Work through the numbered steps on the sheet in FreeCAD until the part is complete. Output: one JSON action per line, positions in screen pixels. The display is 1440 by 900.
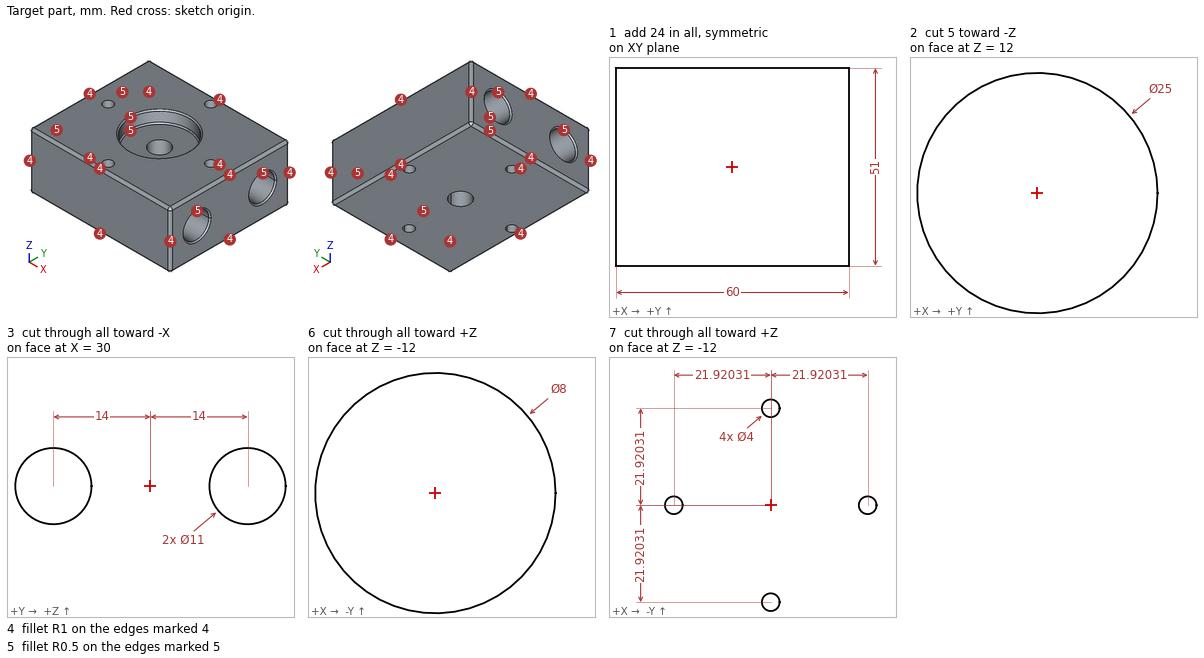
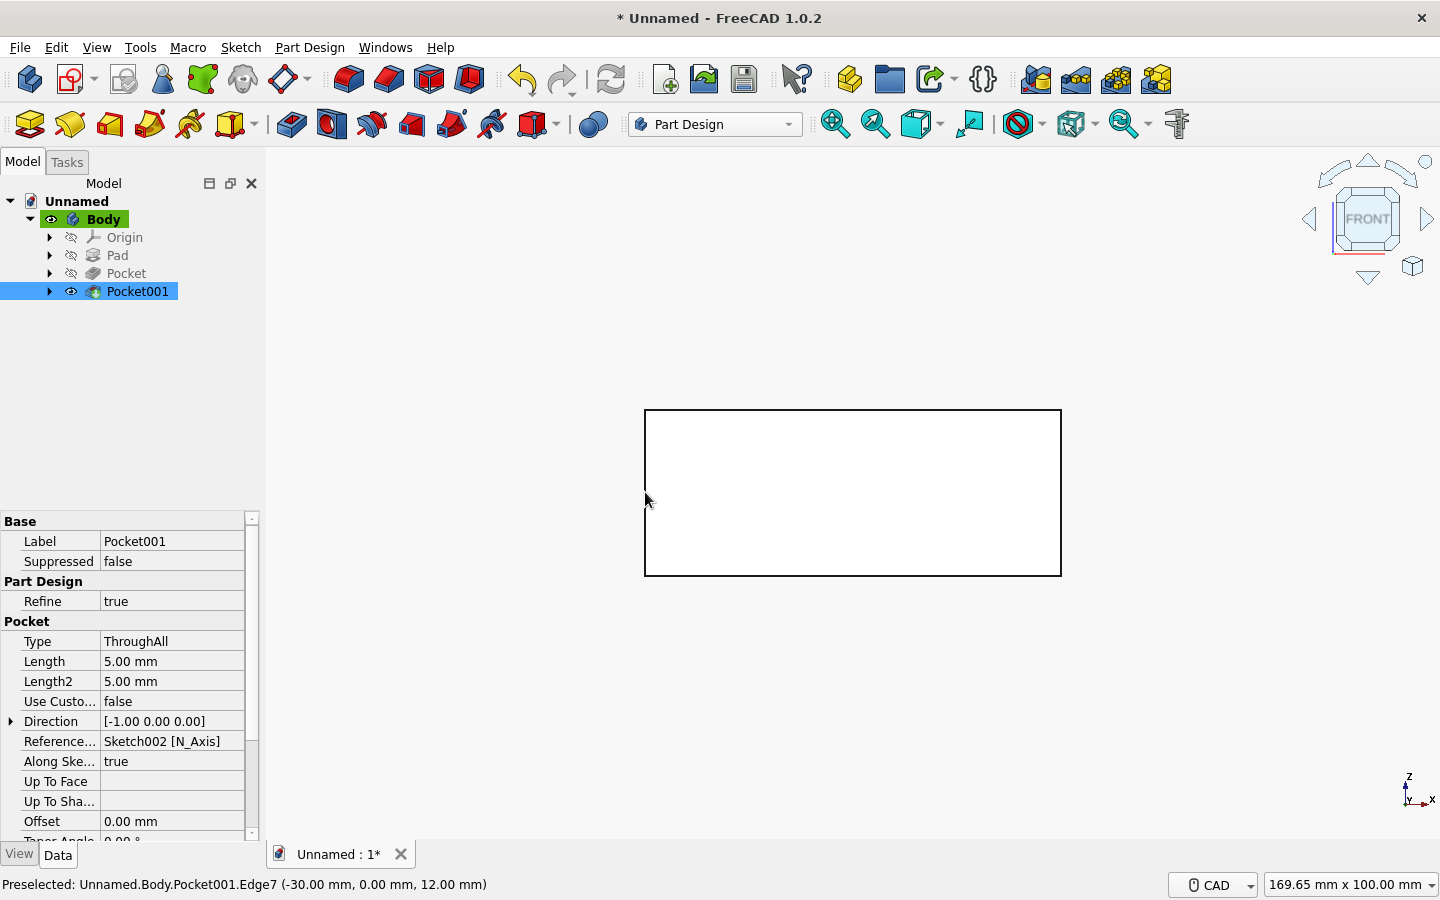
{"action": "key", "text": "v f"}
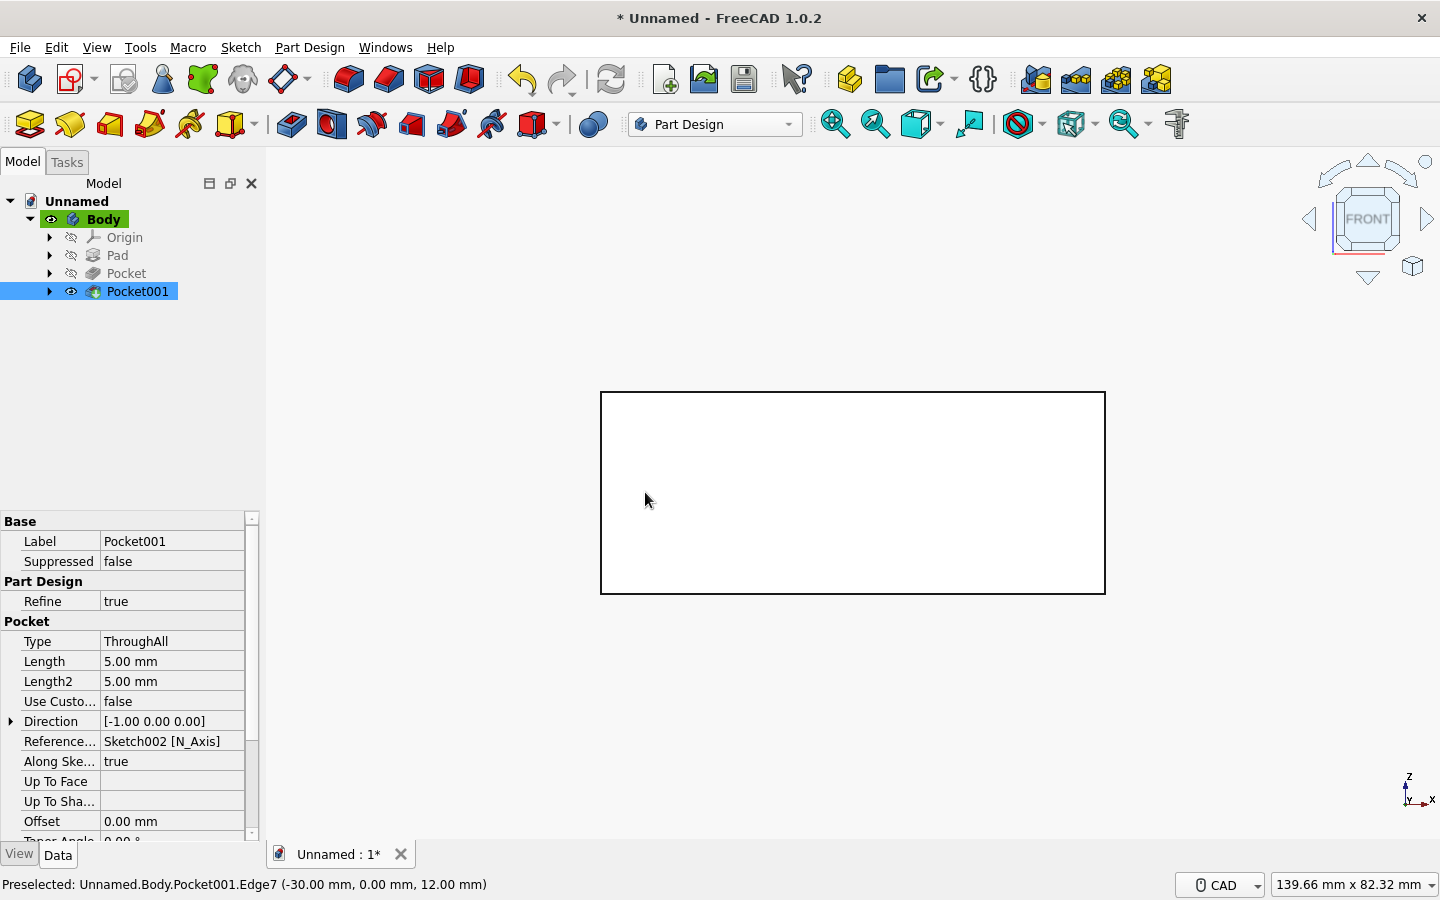
{"action": "key", "text": "3"}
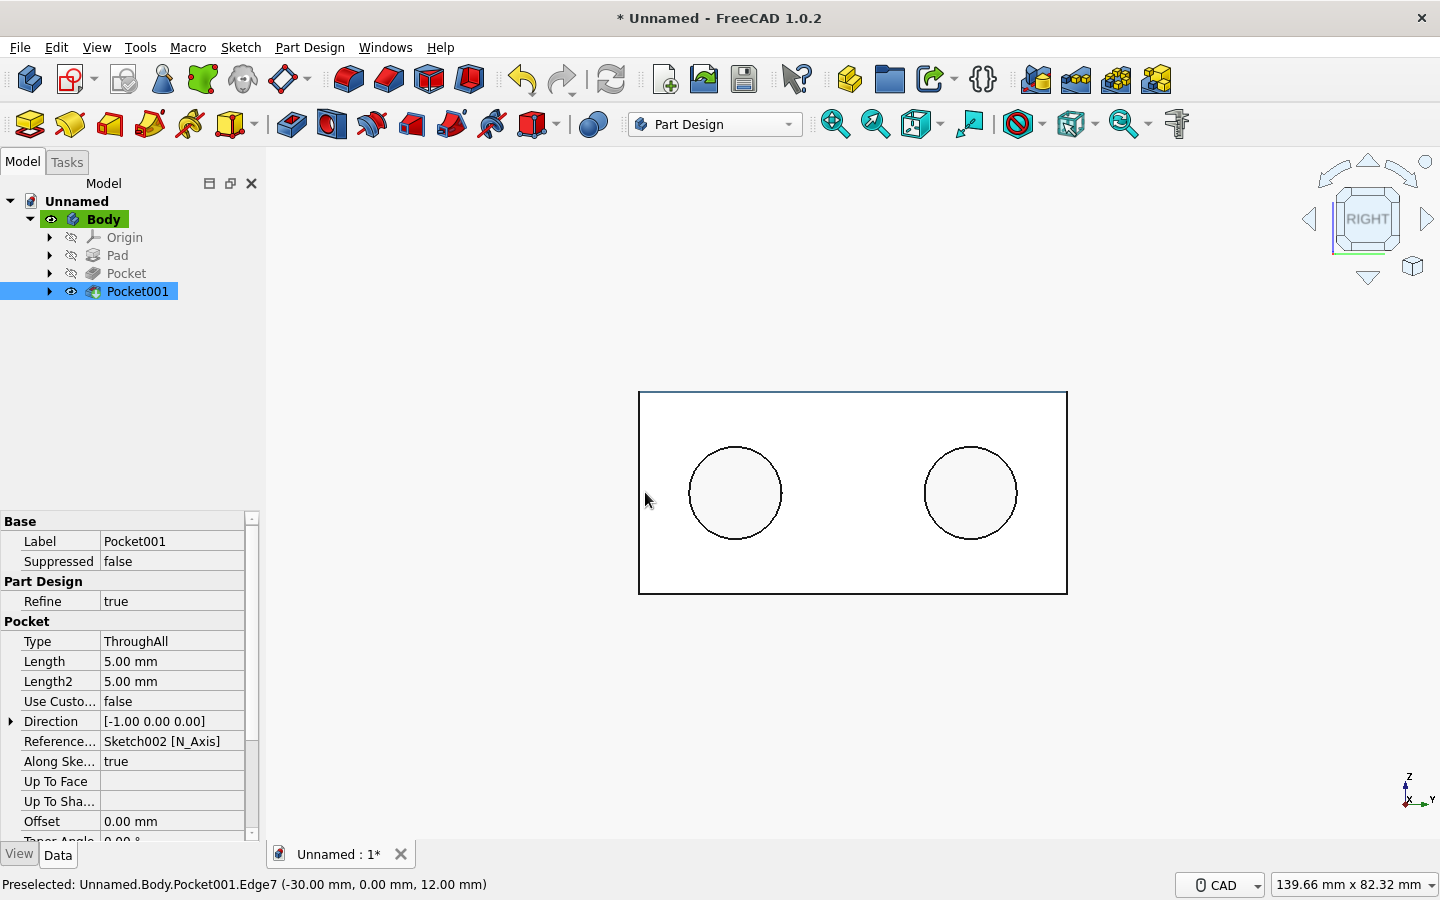
{"action": "key", "text": "v f"}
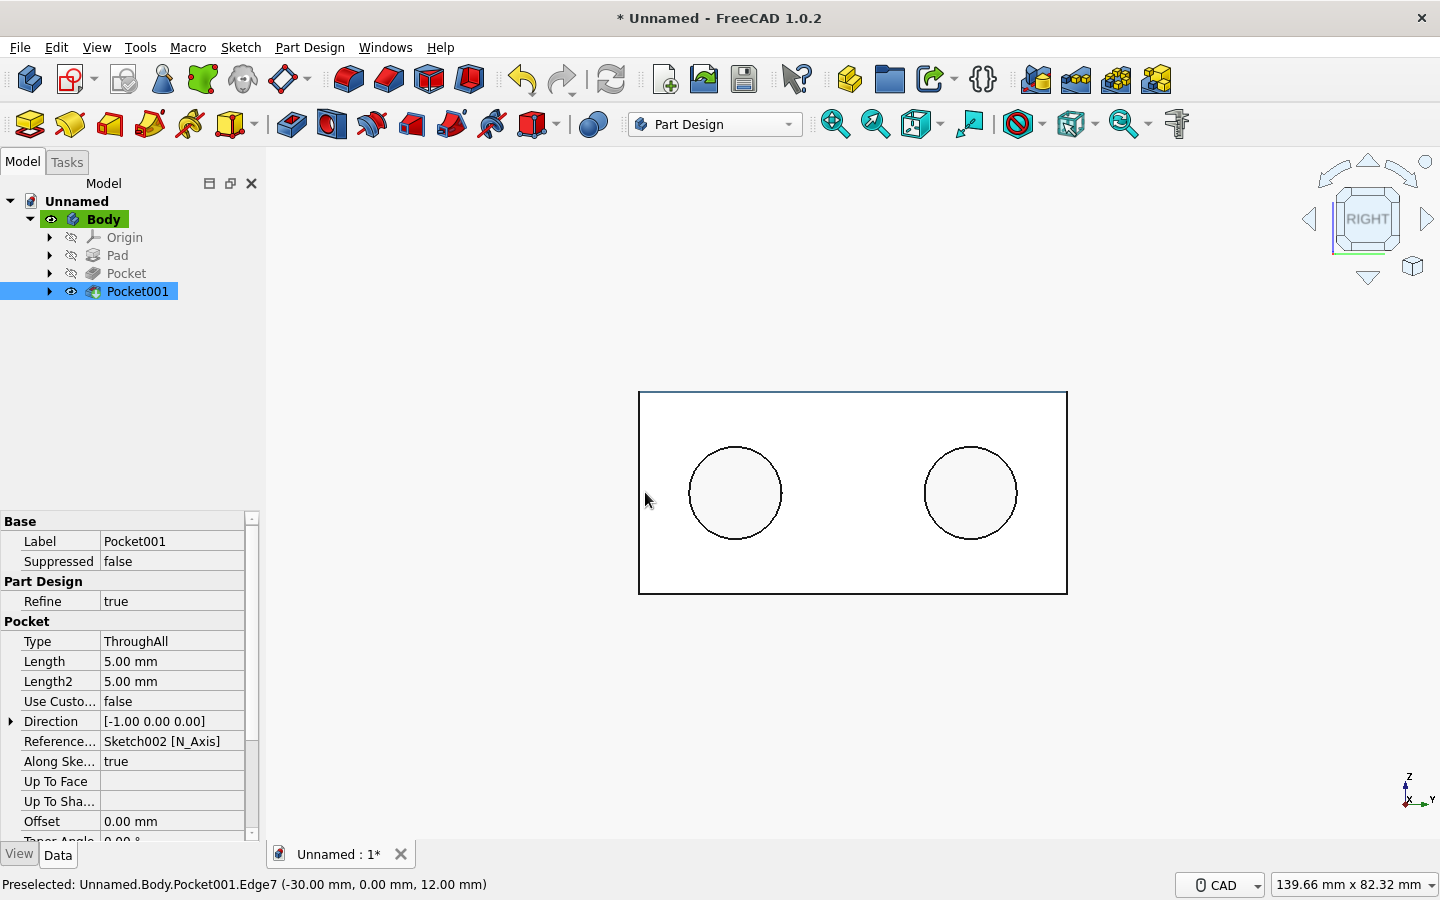
{"action": "key", "text": "5"}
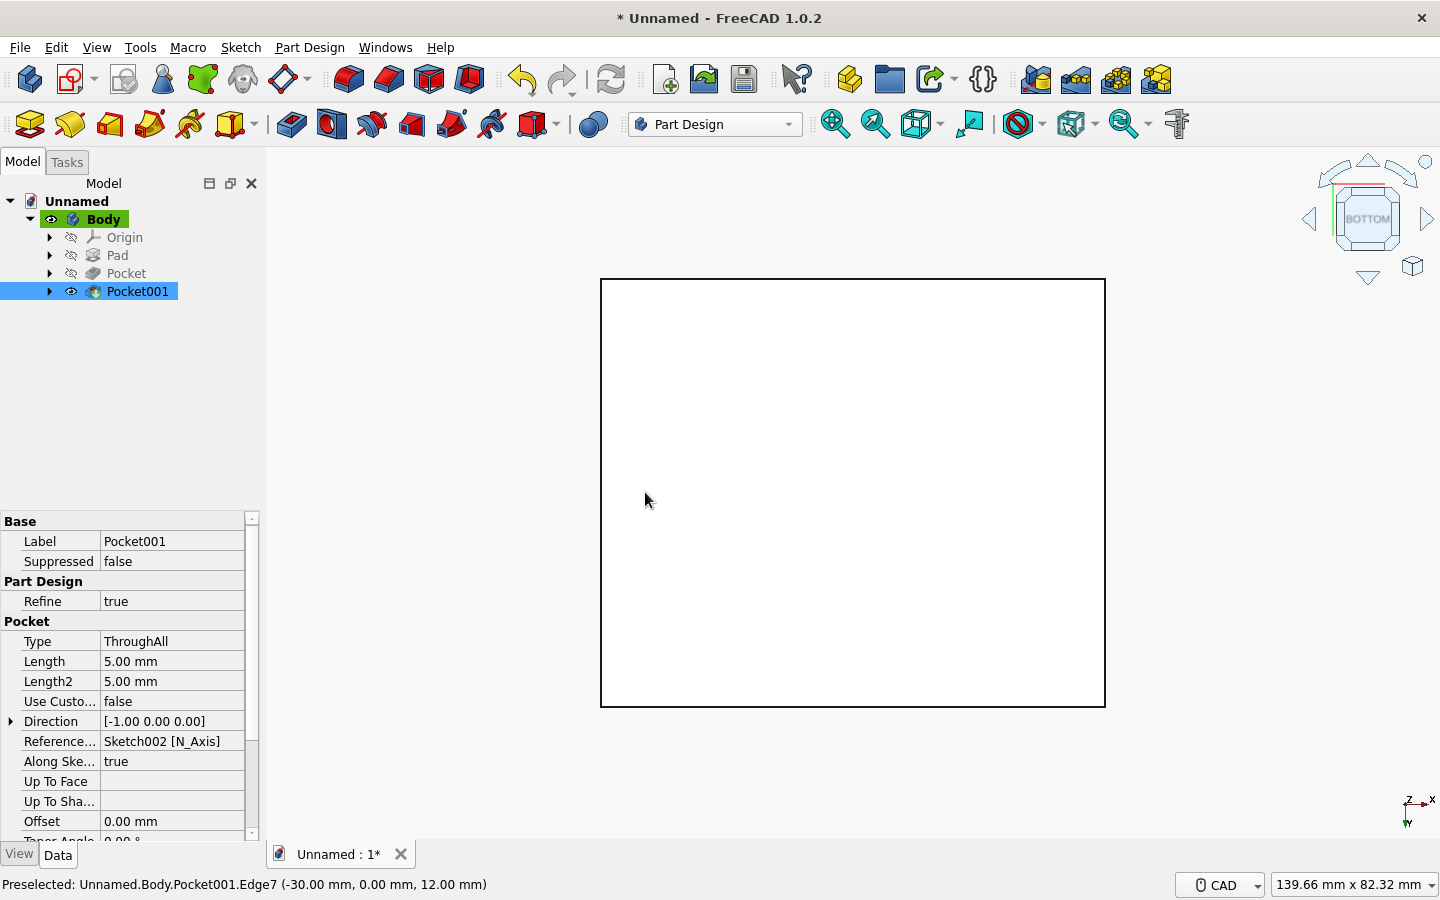
{"action": "left_click", "coordinate": [853, 492], "text": "ctrl"}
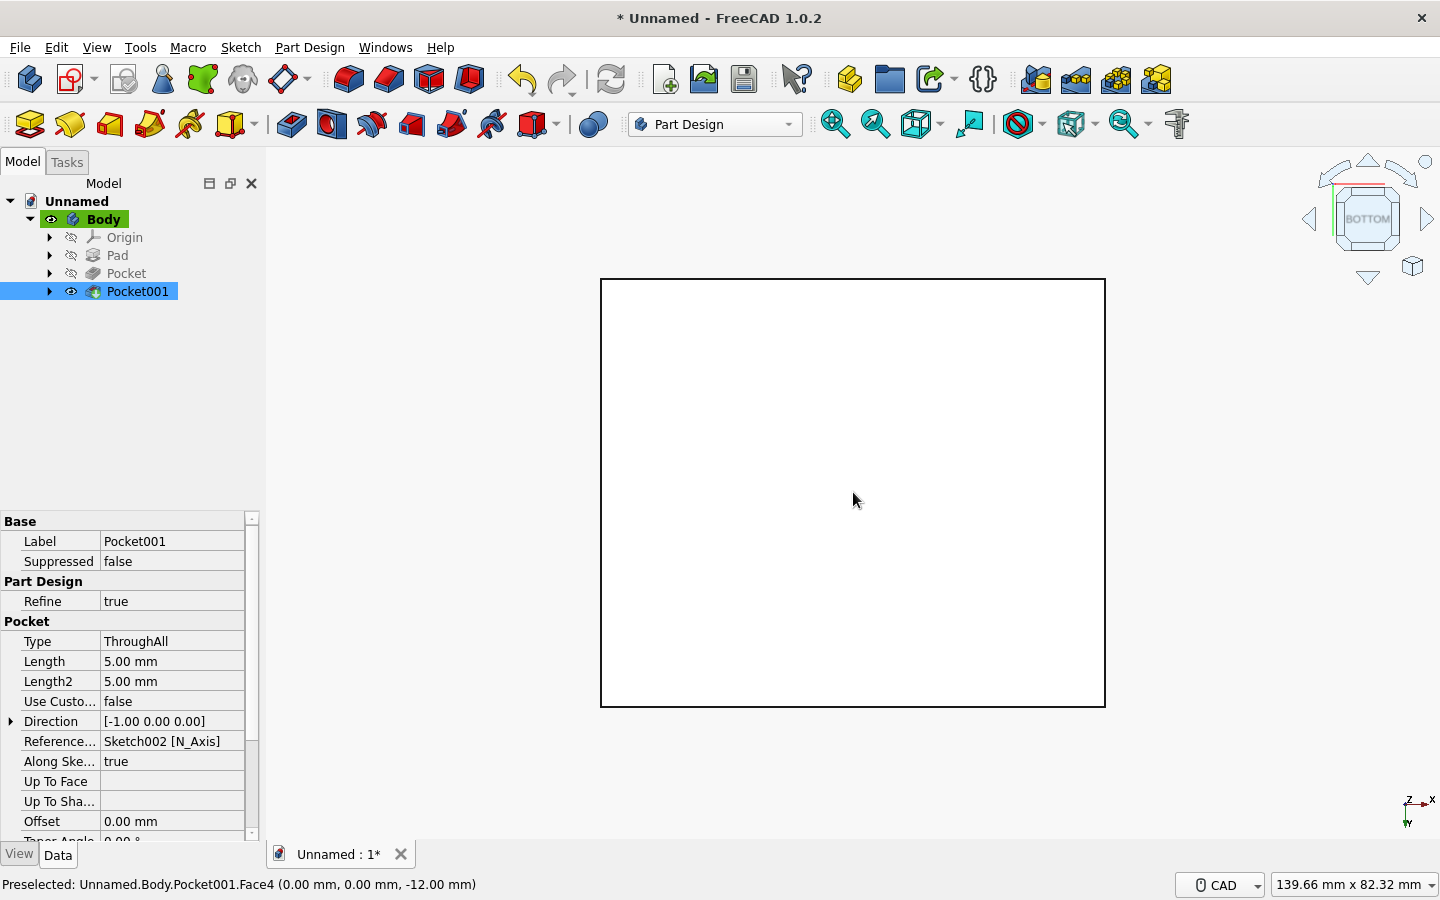
{"action": "key", "text": "4"}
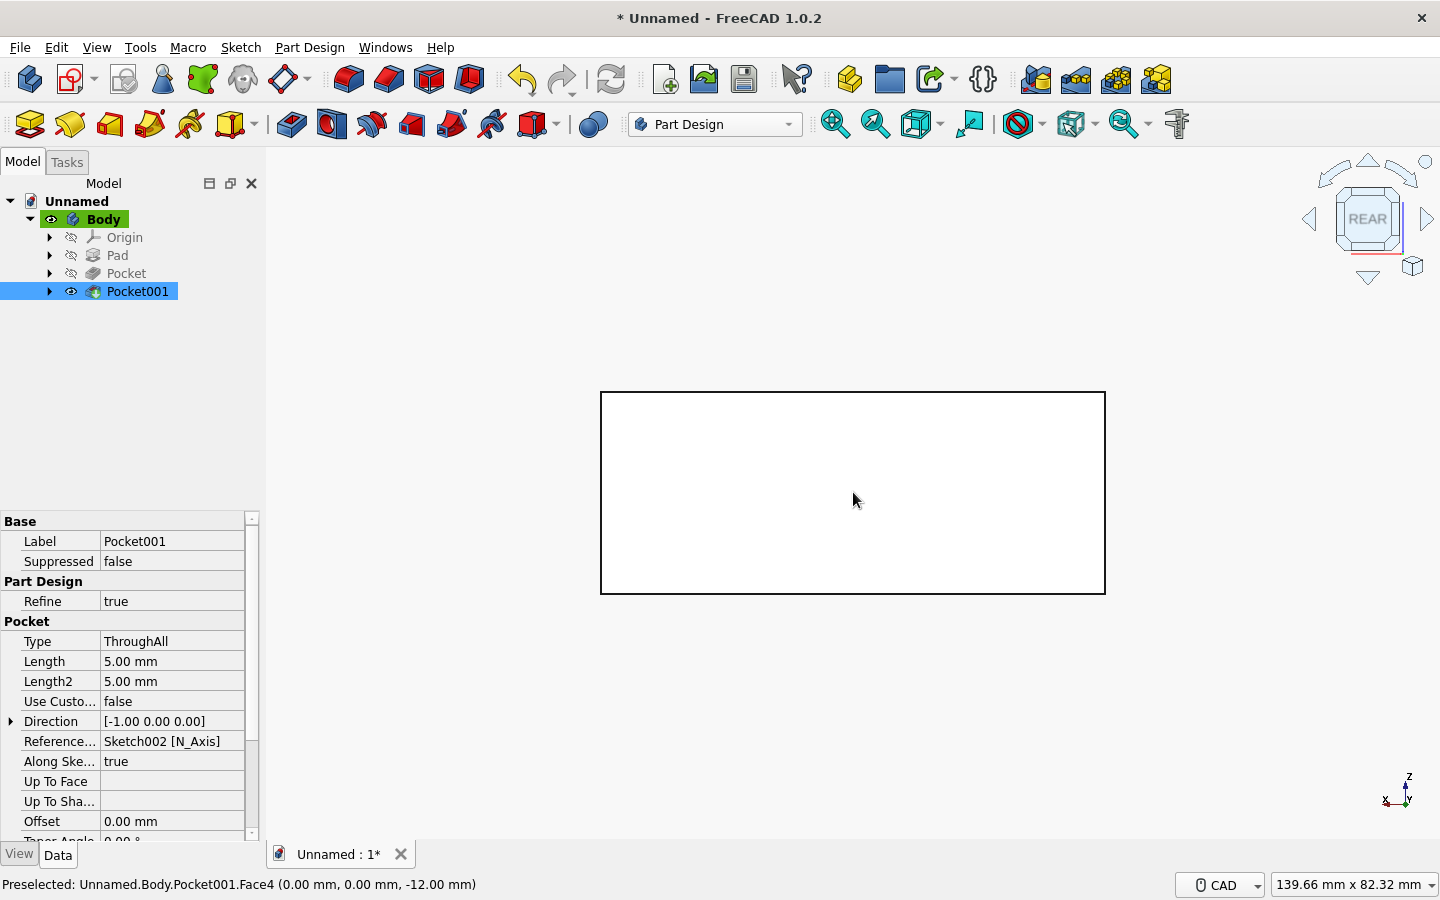
{"action": "left_click", "coordinate": [836, 124]}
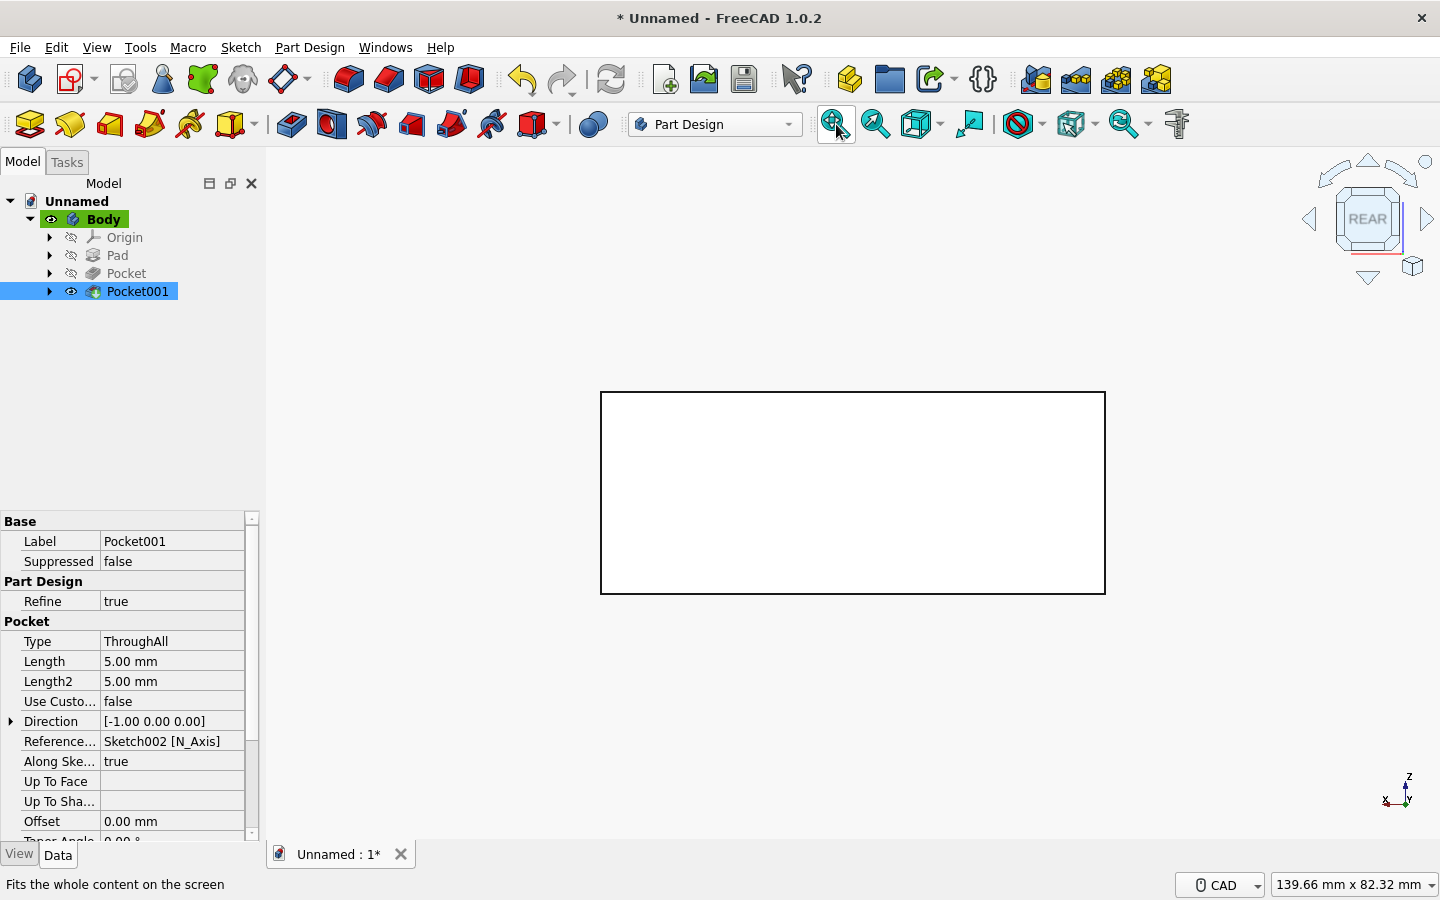
{"action": "left_click", "coordinate": [709, 492], "text": "ctrl"}